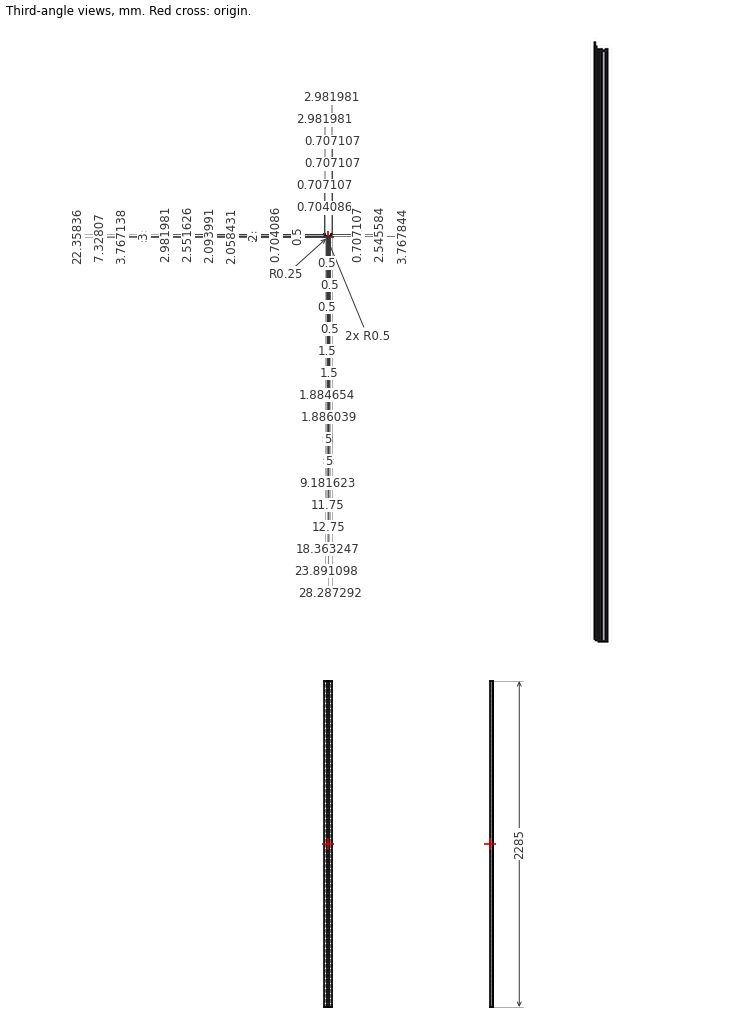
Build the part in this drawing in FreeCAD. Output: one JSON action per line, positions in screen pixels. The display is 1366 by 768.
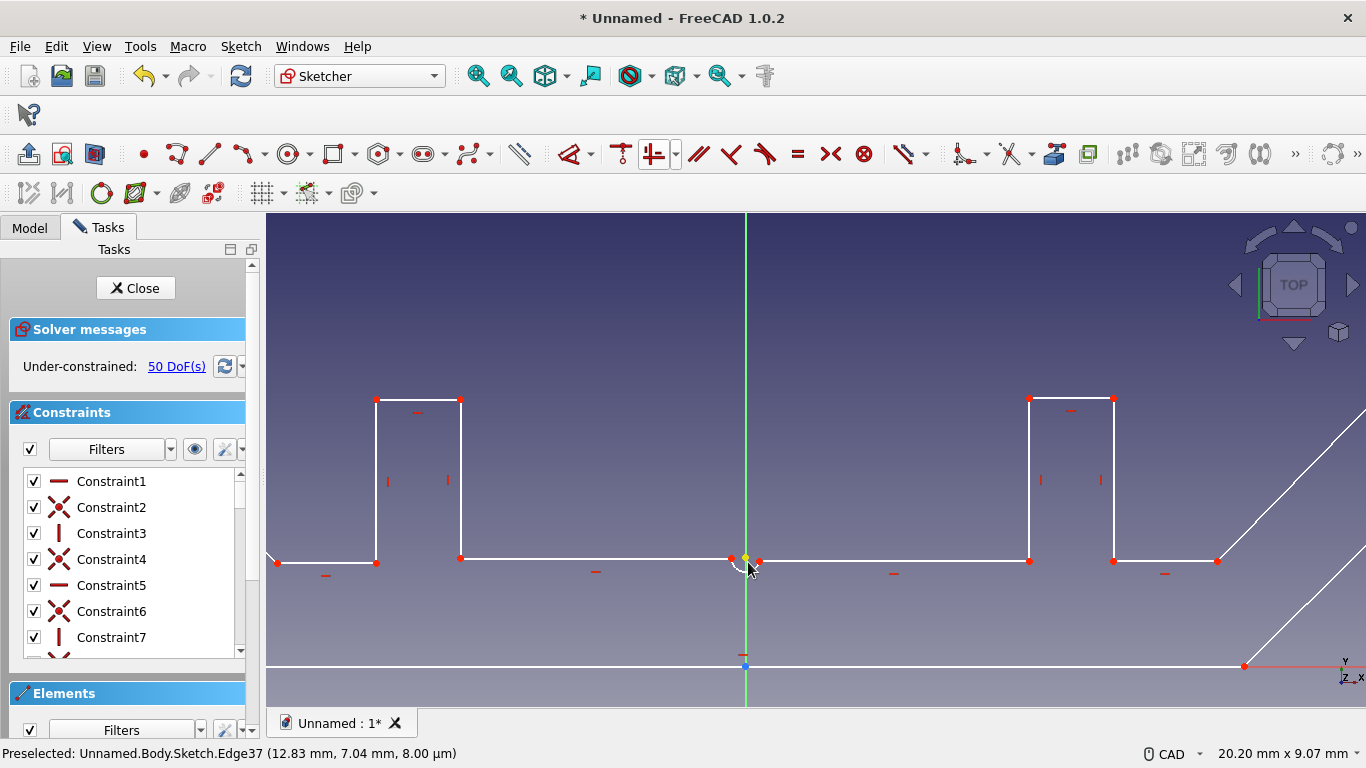
{"action": "left_click", "coordinate": [746, 558]}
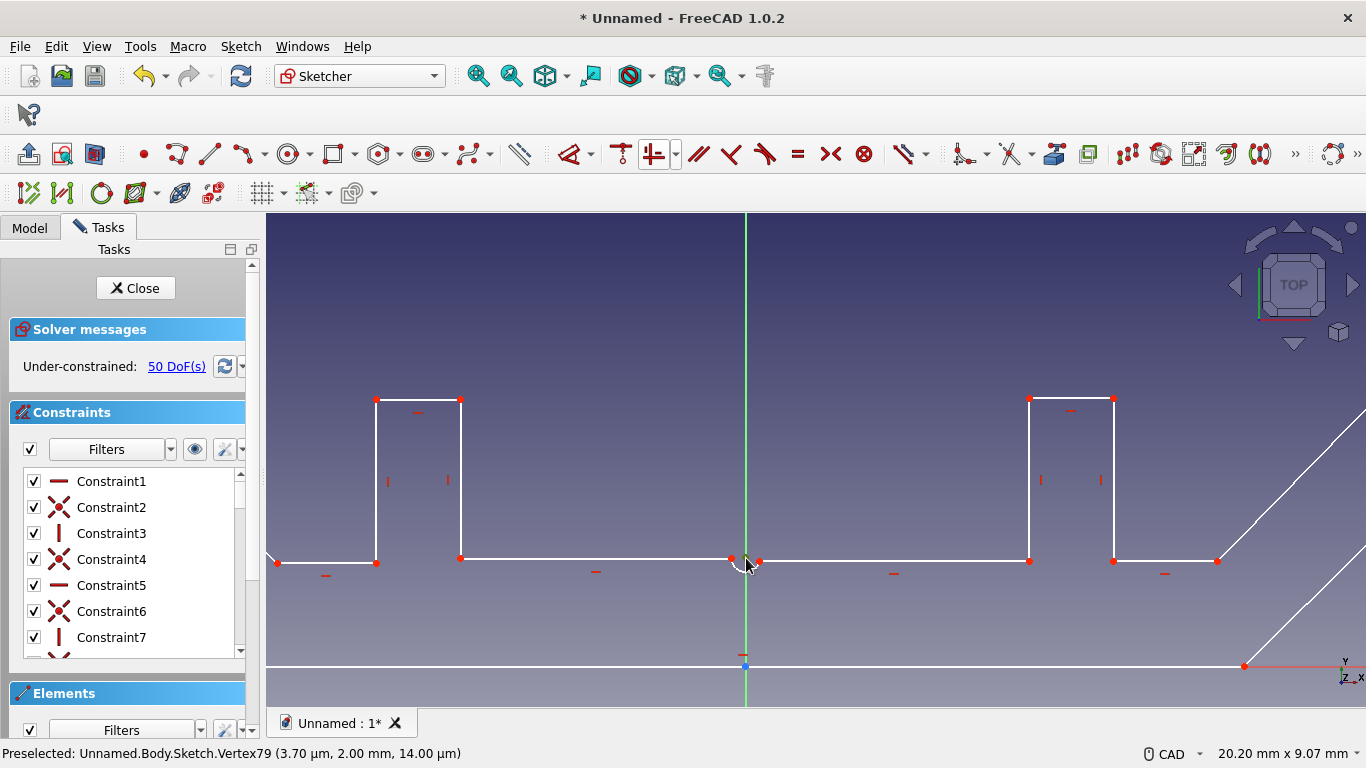
{"action": "left_click", "coordinate": [746, 616]}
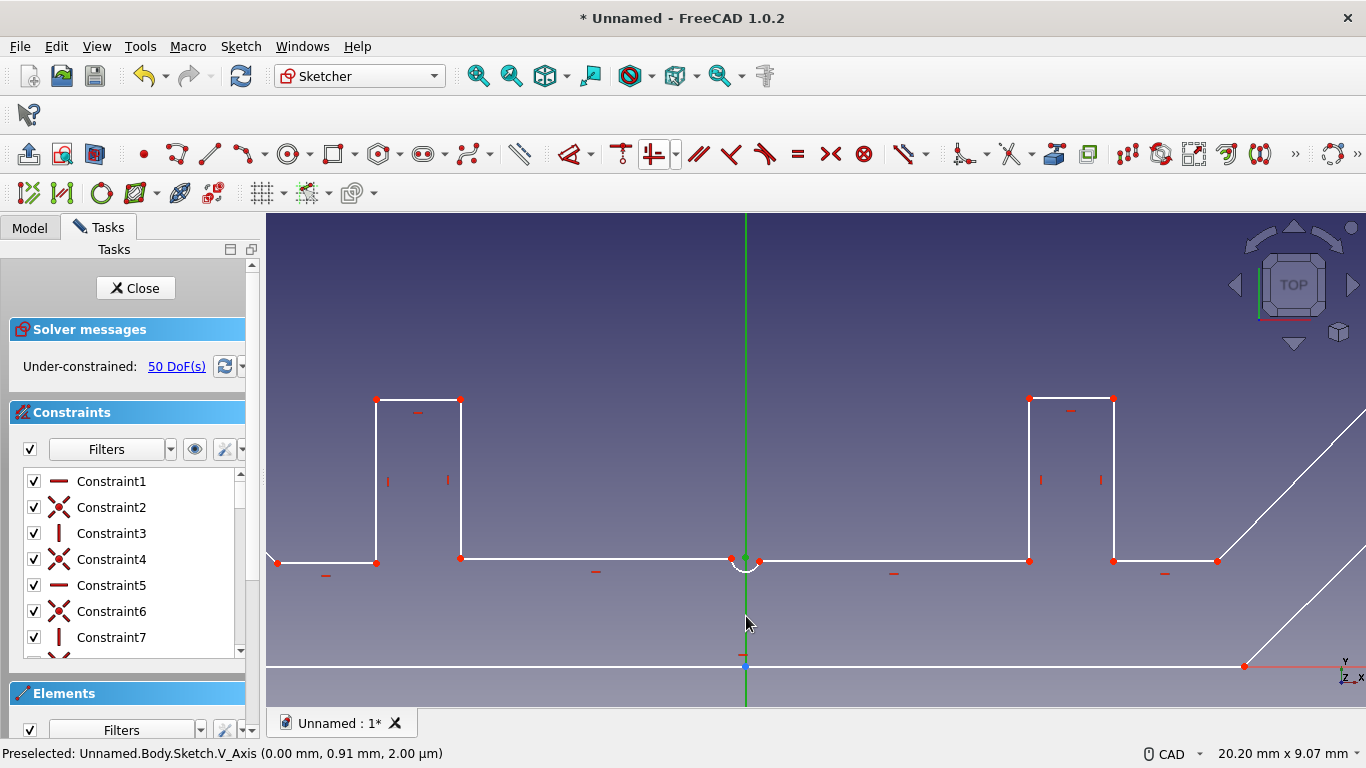
{"action": "left_click", "coordinate": [621, 154]}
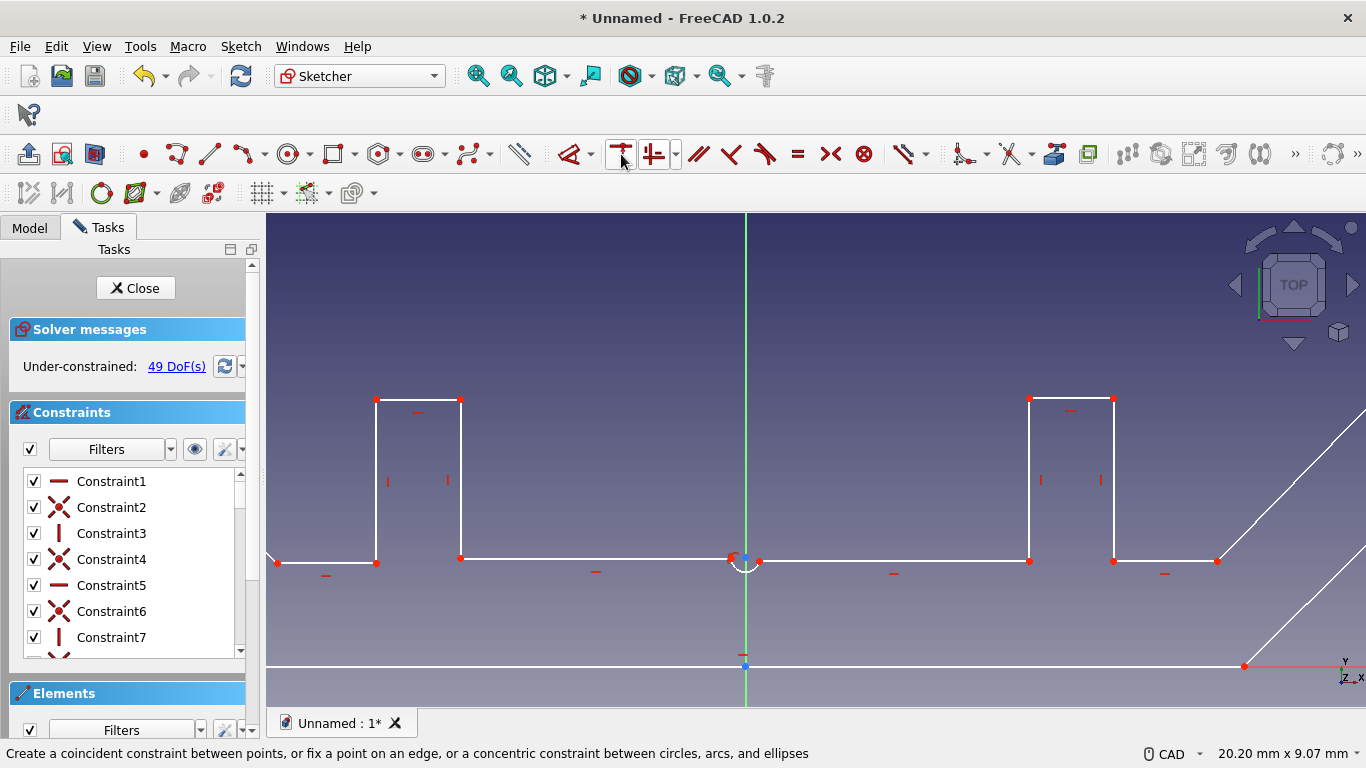
{"action": "left_click", "coordinate": [568, 154]}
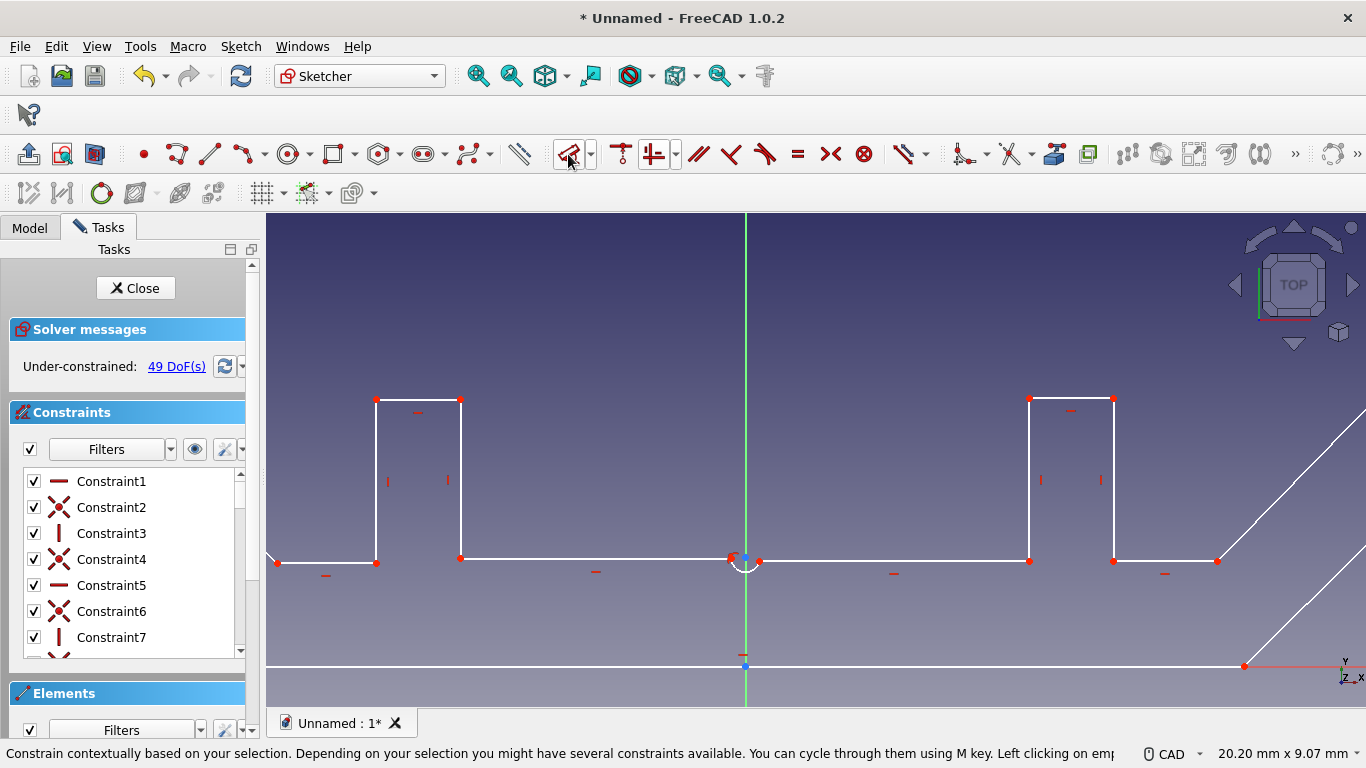
{"action": "scroll", "coordinate": [748, 562], "scroll_direction": "down", "scroll_amount": 8}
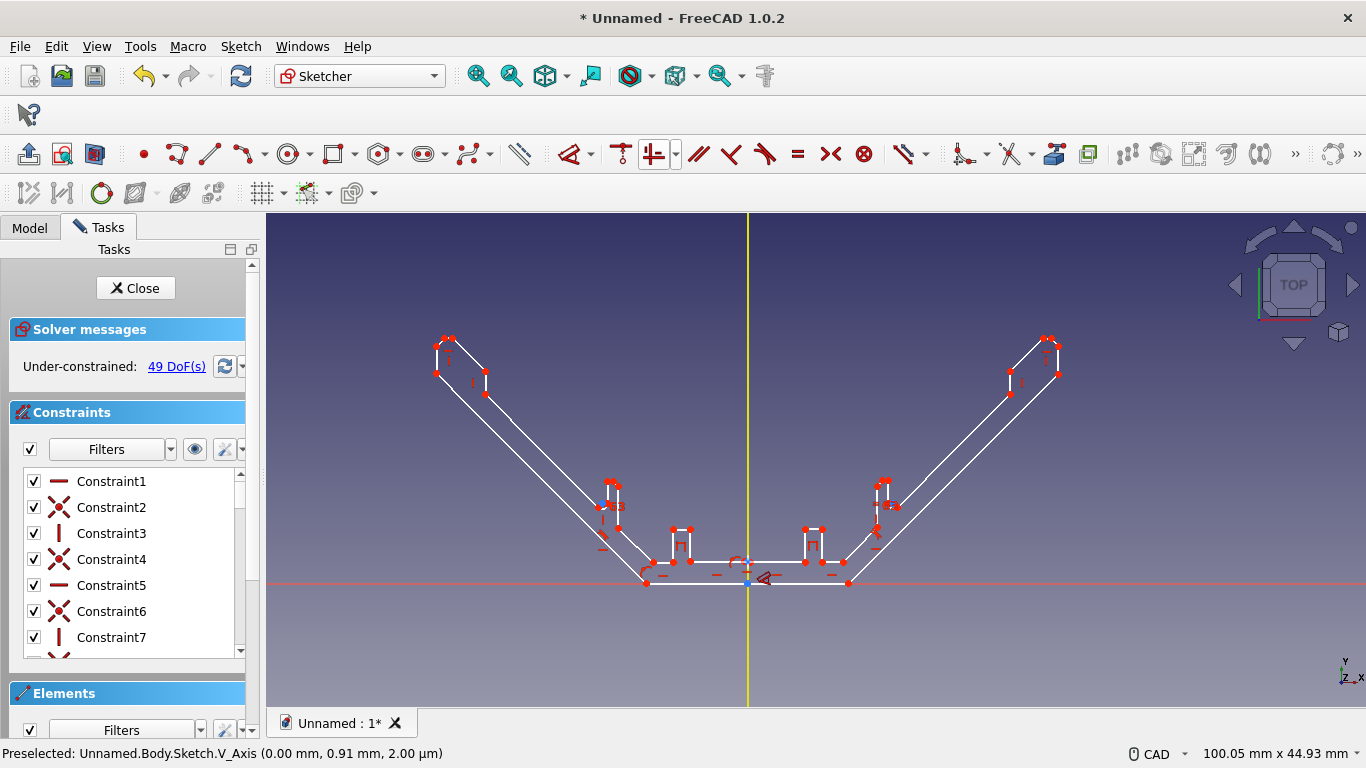
{"action": "scroll", "coordinate": [602, 509], "scroll_direction": "up", "scroll_amount": 10}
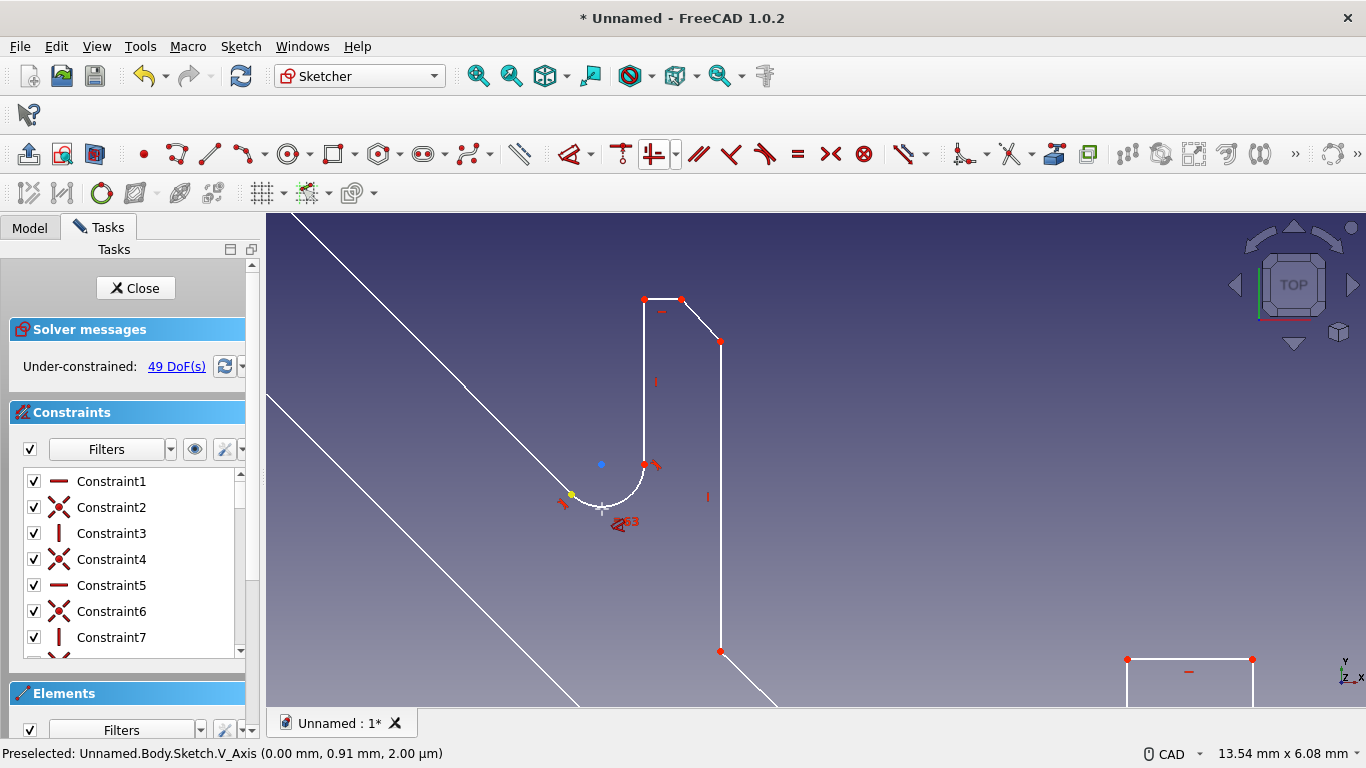
{"action": "left_click", "coordinate": [598, 507]}
{"action": "left_click", "coordinate": [595, 539]}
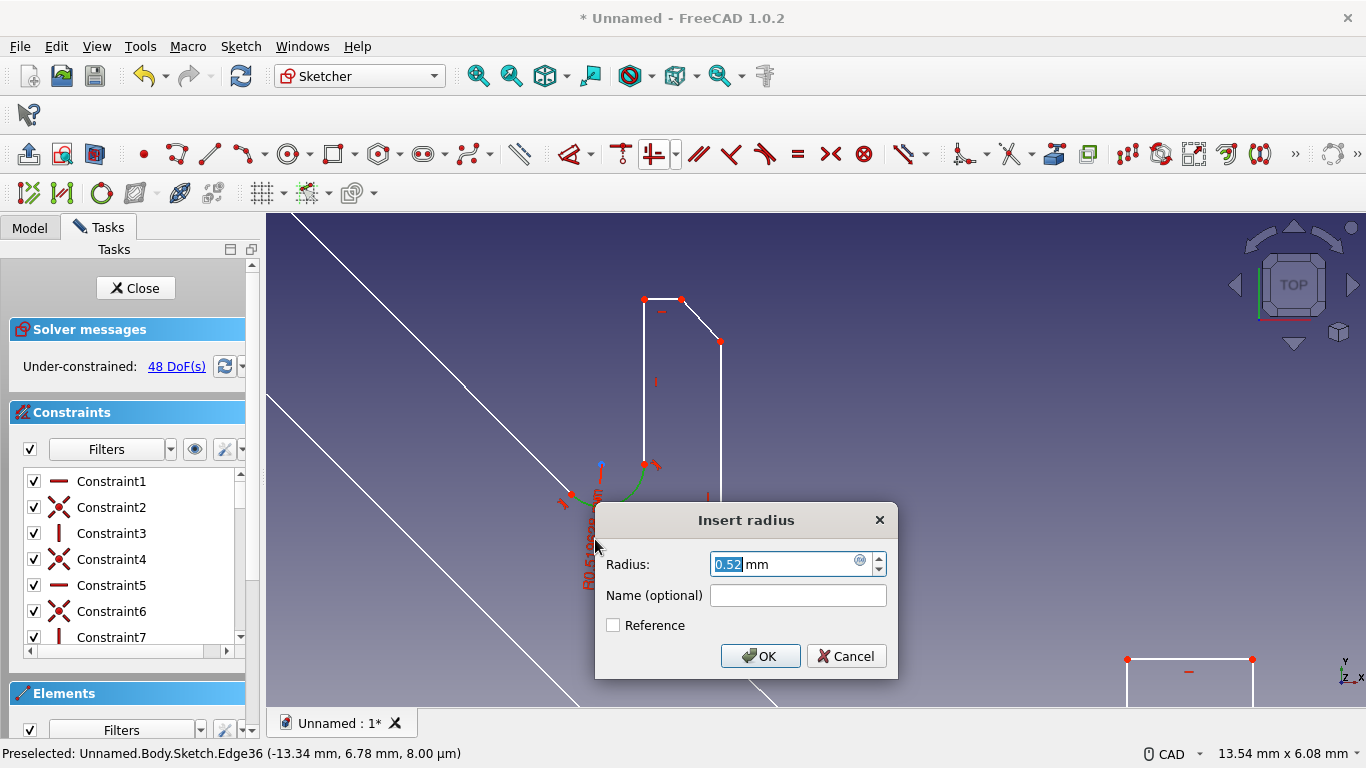
{"action": "type", "text": "0.5"}
{"action": "key", "text": "Return"}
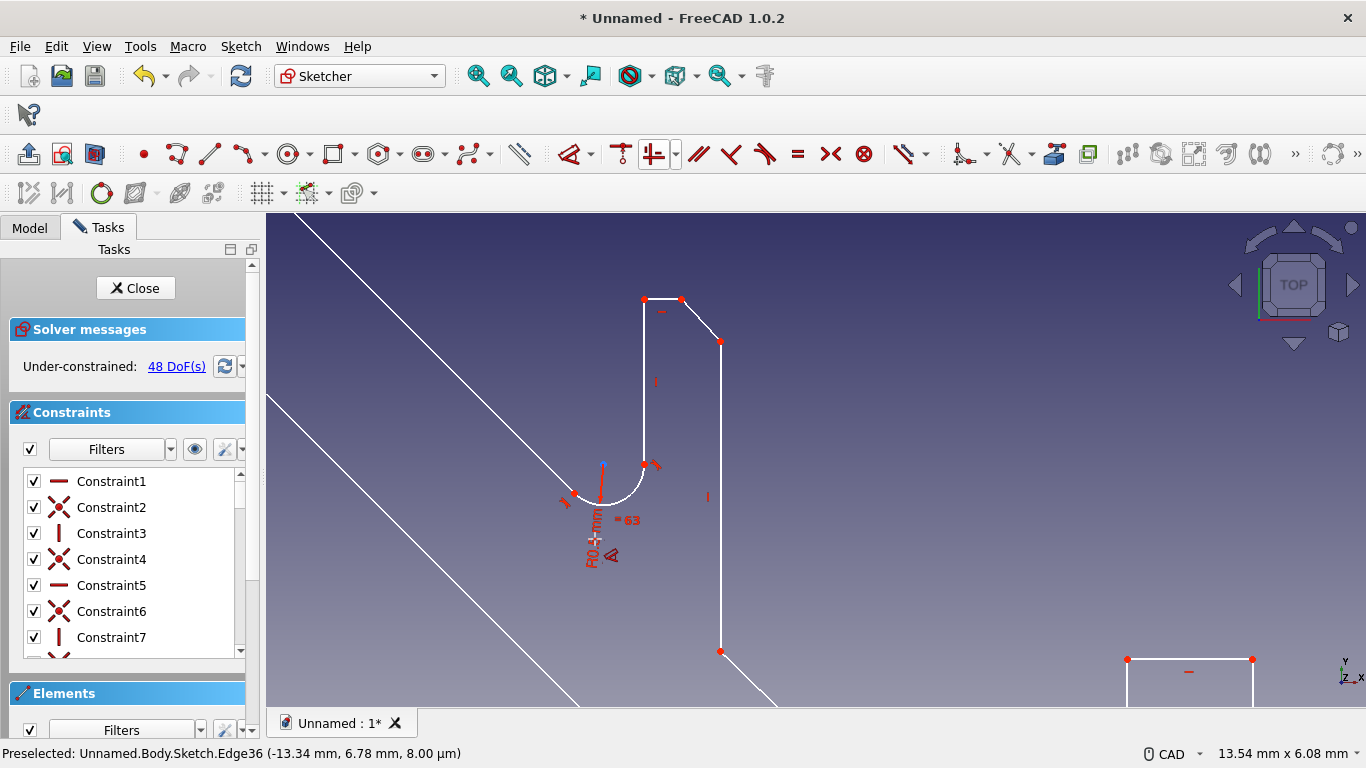
{"action": "scroll", "coordinate": [602, 509], "scroll_direction": "down", "scroll_amount": 10}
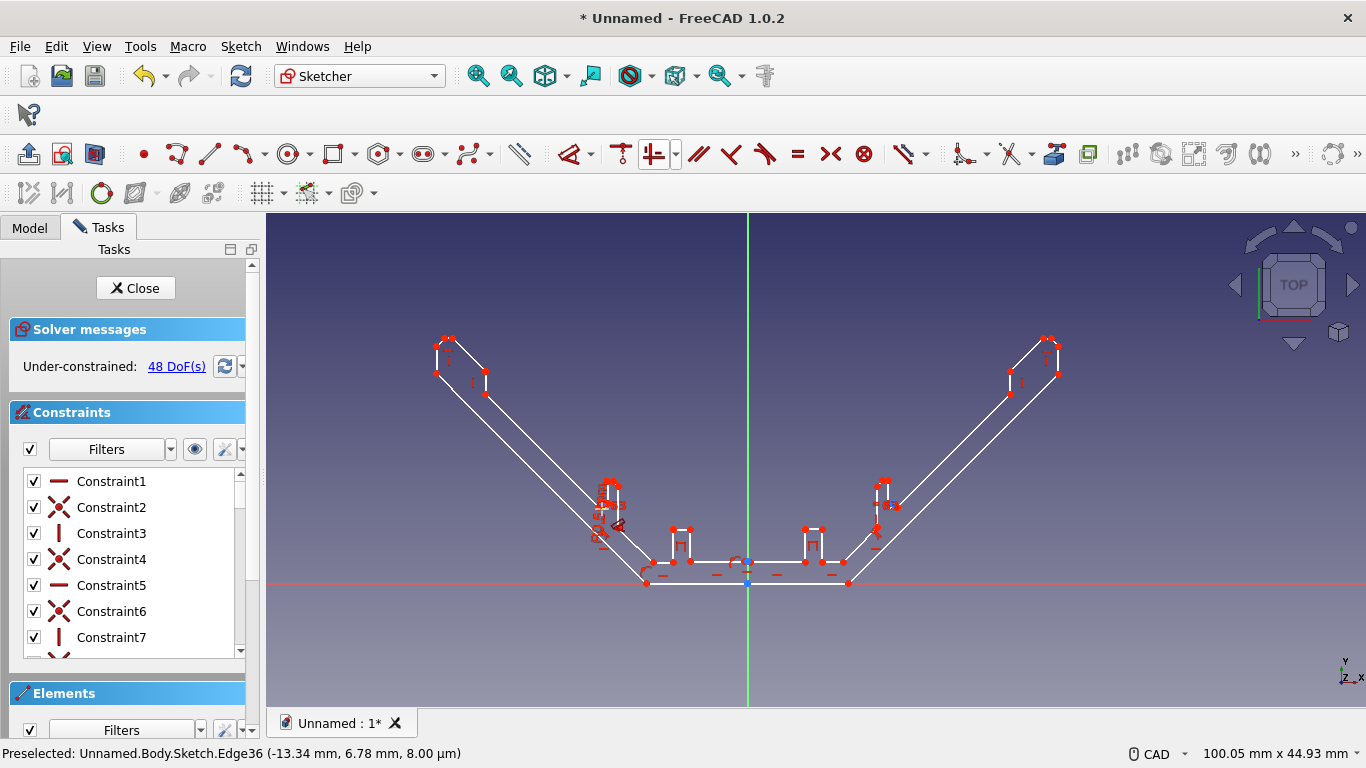
{"action": "scroll", "coordinate": [746, 564], "scroll_direction": "up", "scroll_amount": 14}